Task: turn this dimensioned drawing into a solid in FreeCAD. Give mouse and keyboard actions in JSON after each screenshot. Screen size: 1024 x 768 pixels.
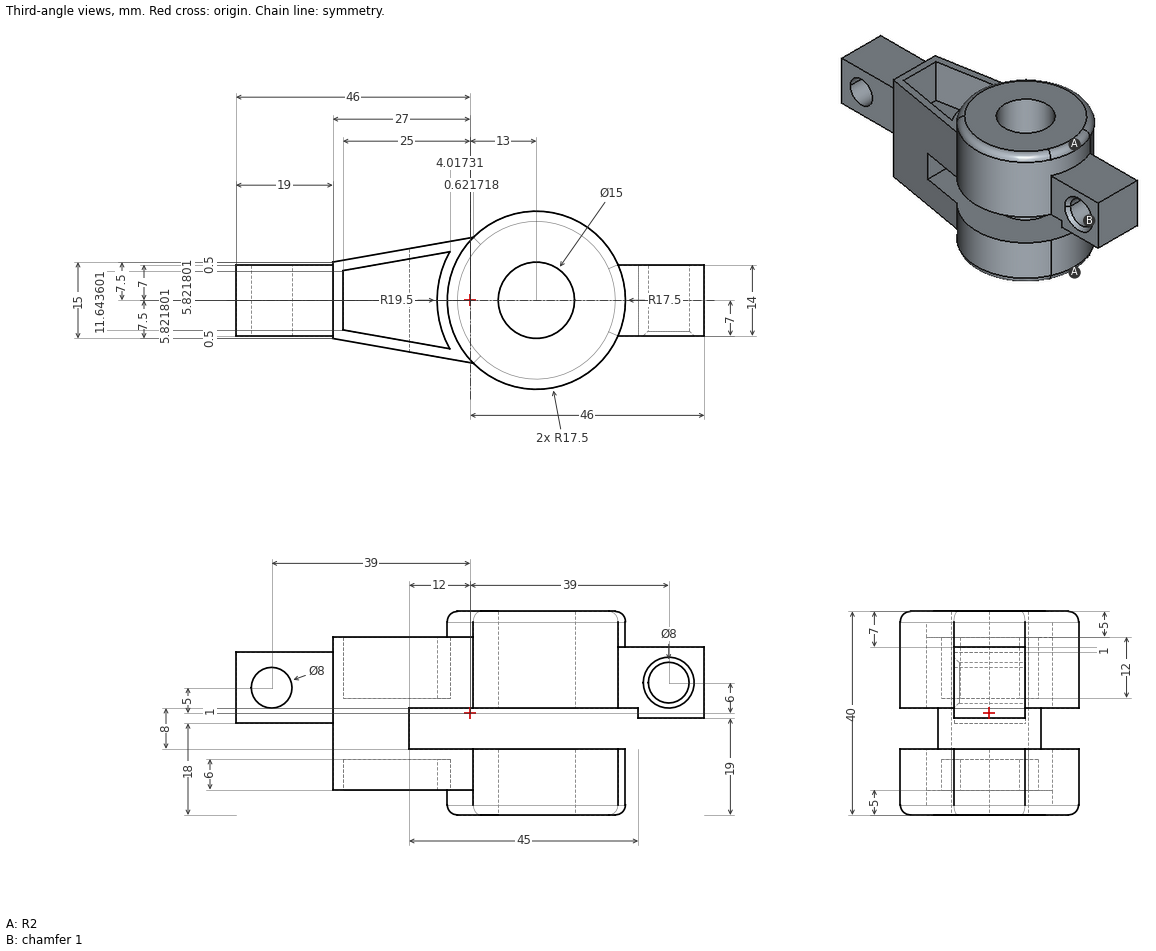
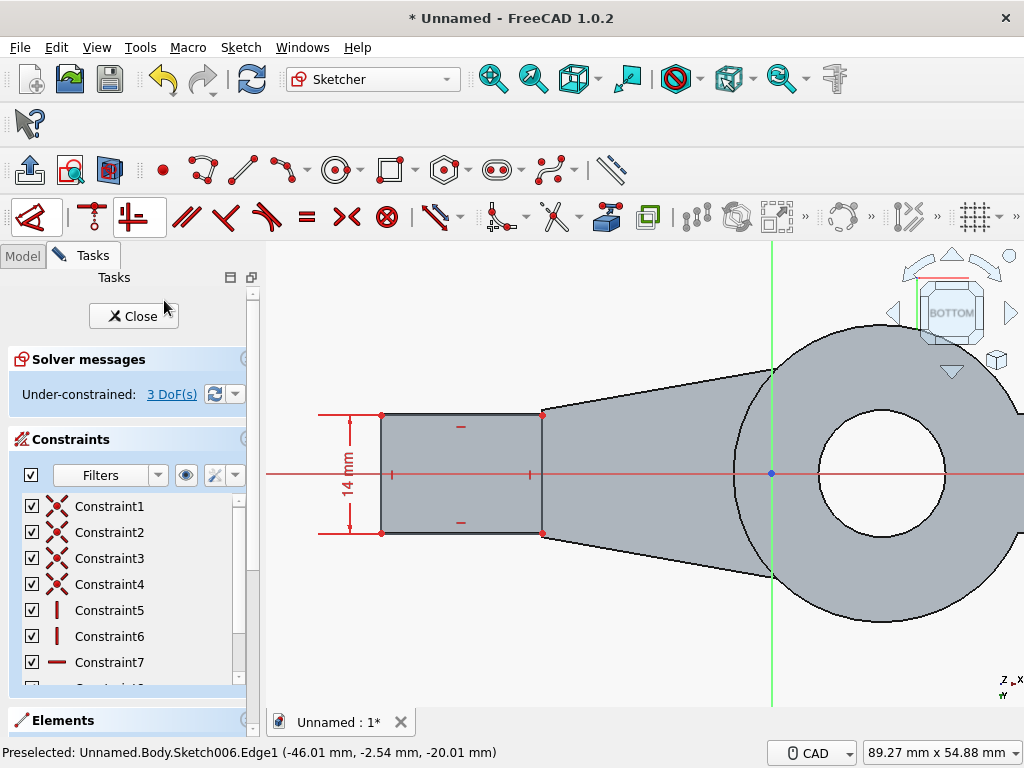
{"action": "left_click", "coordinate": [429, 534]}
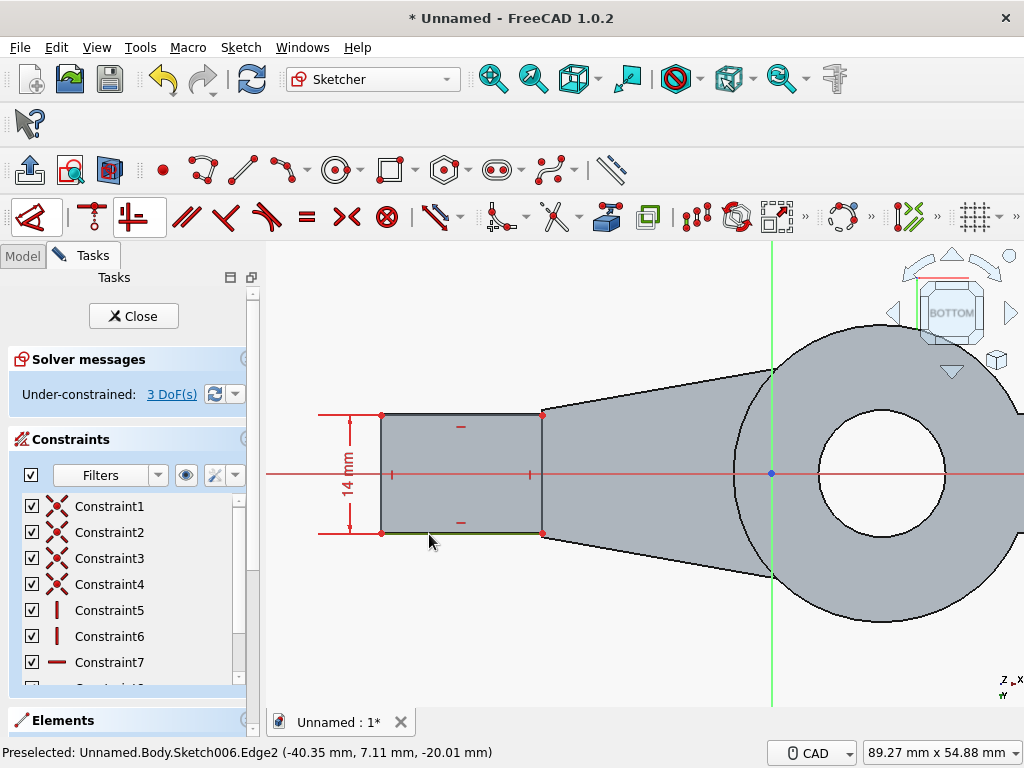
{"action": "left_click", "coordinate": [56, 218]}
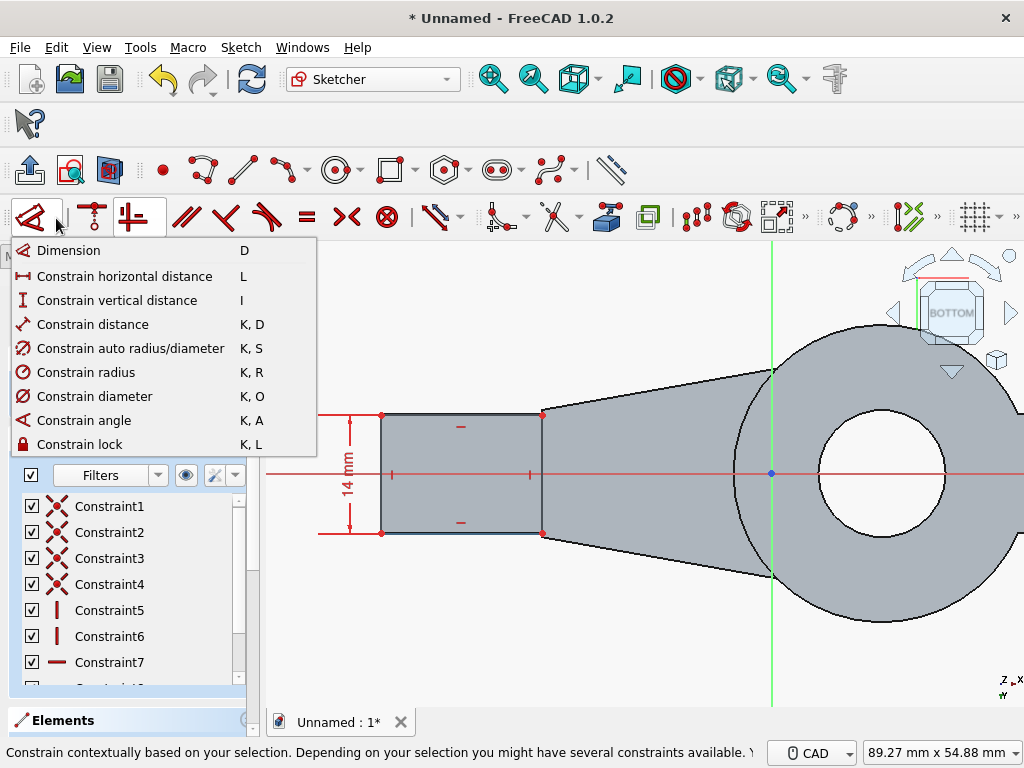
{"action": "left_click", "coordinate": [164, 276]}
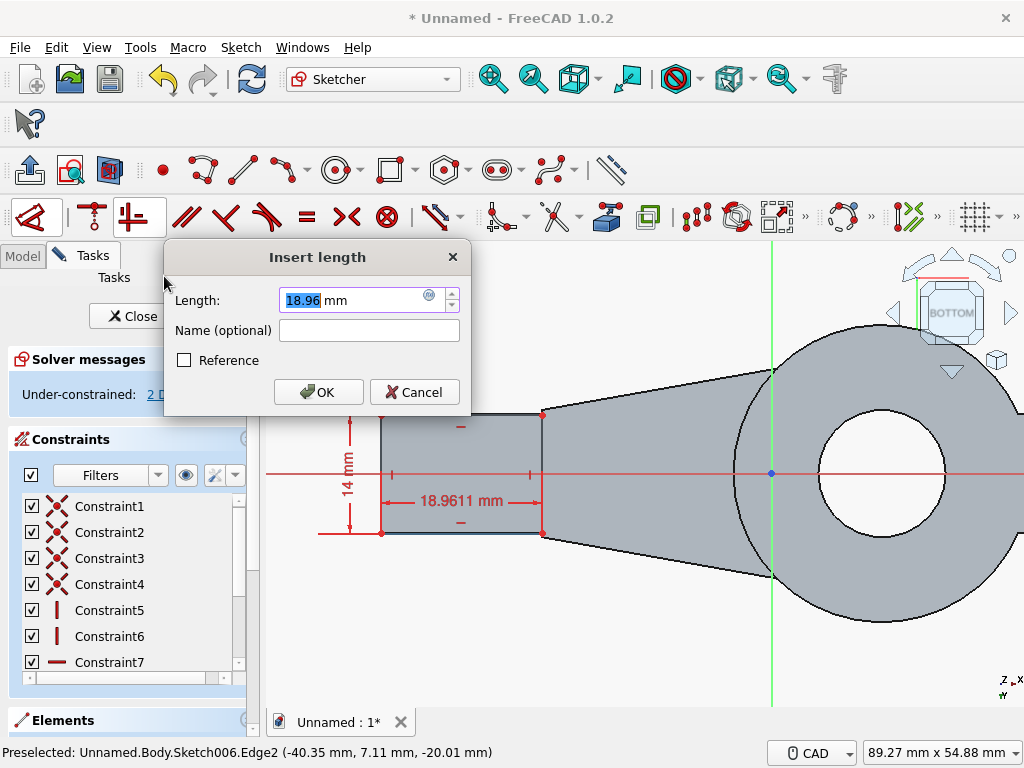
{"action": "type", "text": "19"}
{"action": "key", "text": "Return"}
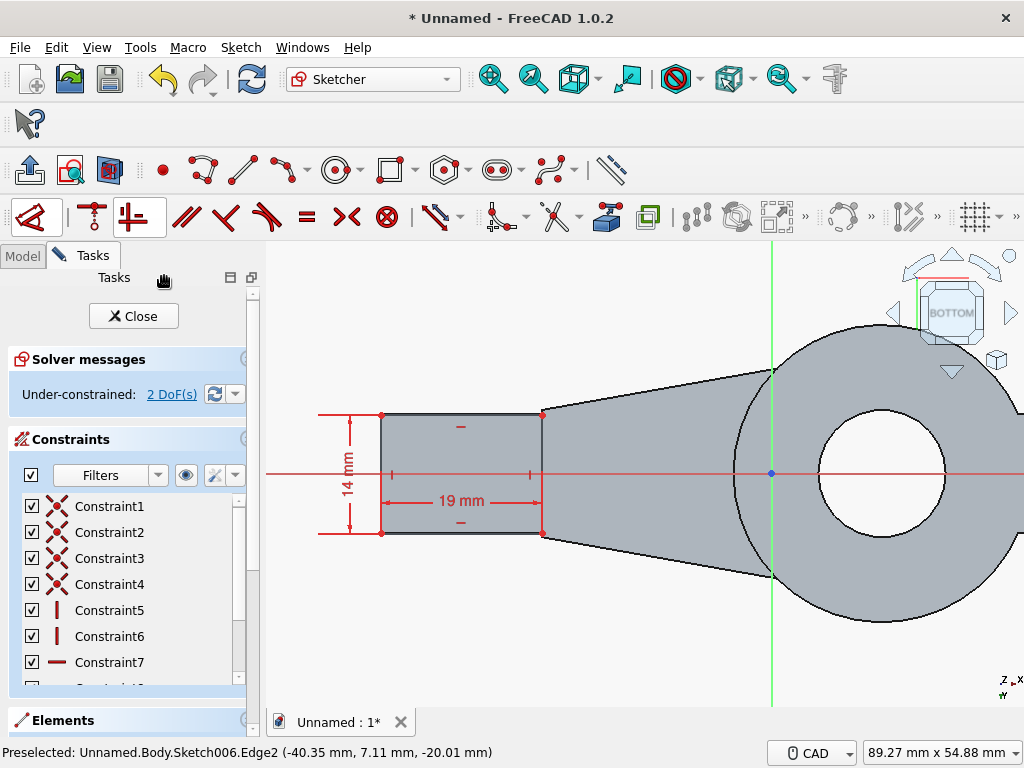
{"action": "left_click", "coordinate": [381, 415]}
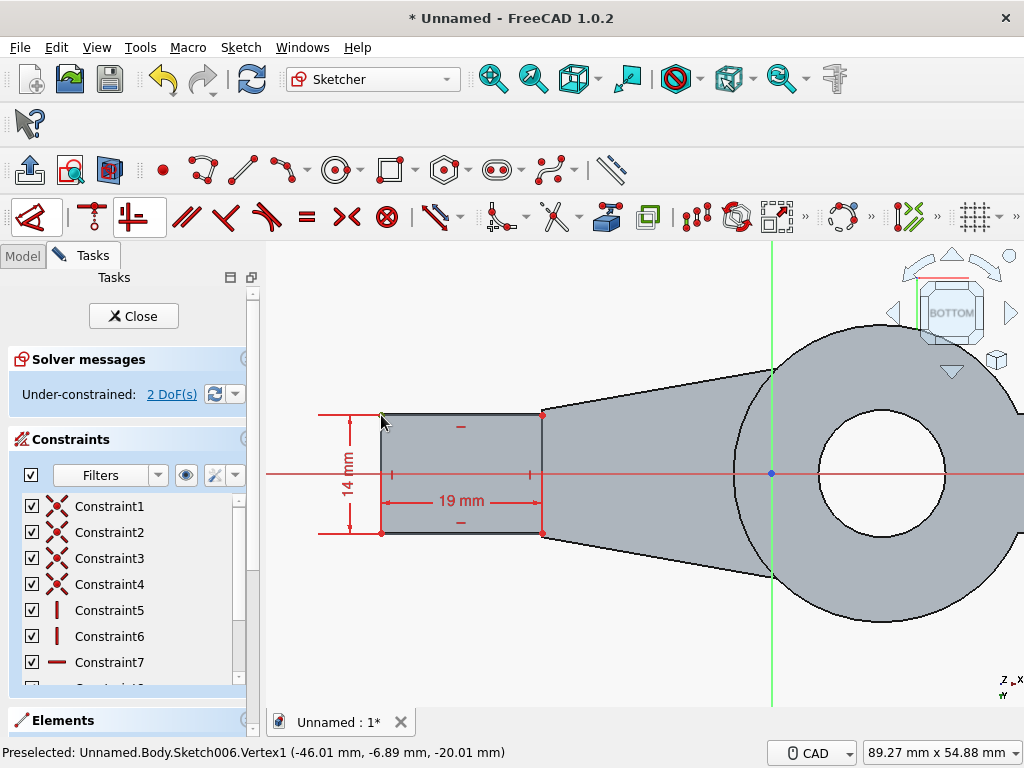
{"action": "left_click", "coordinate": [56, 218]}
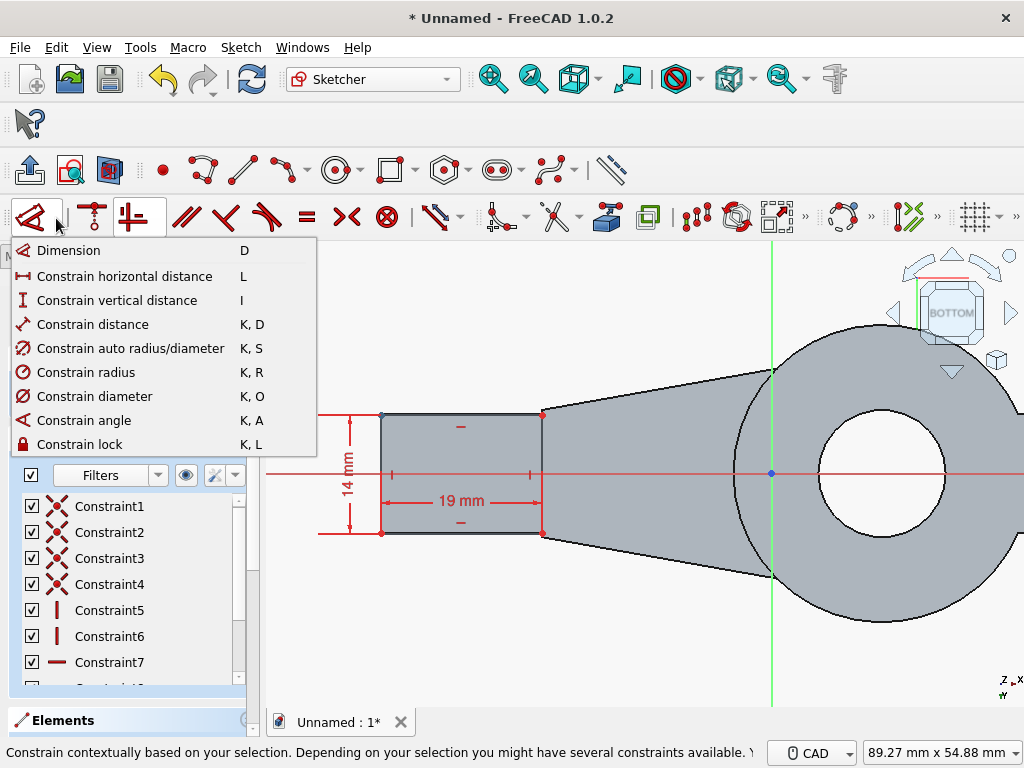
{"action": "left_click", "coordinate": [164, 300]}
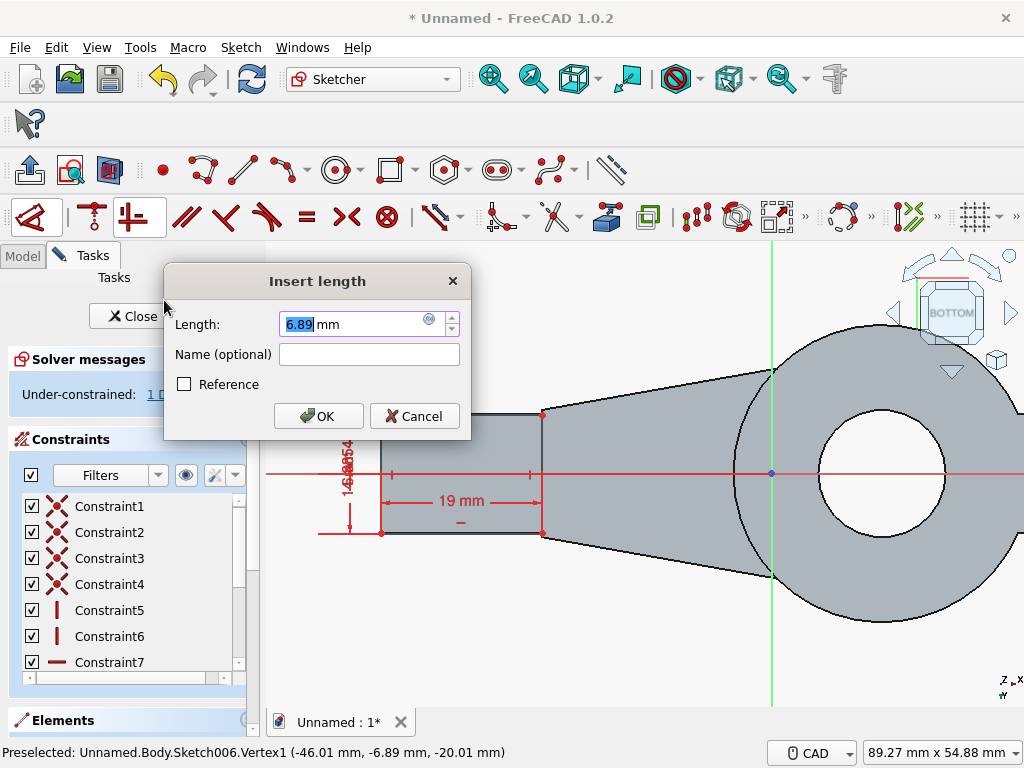
{"action": "type", "text": "7"}
{"action": "key", "text": "Return"}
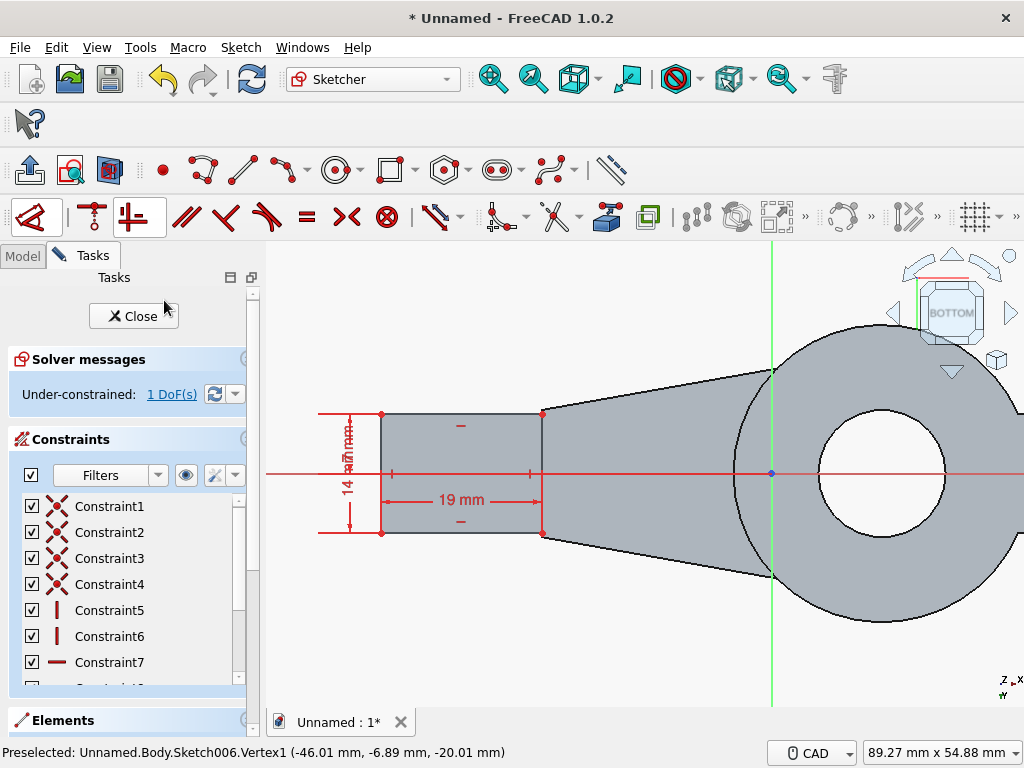
{"action": "left_click", "coordinate": [381, 414]}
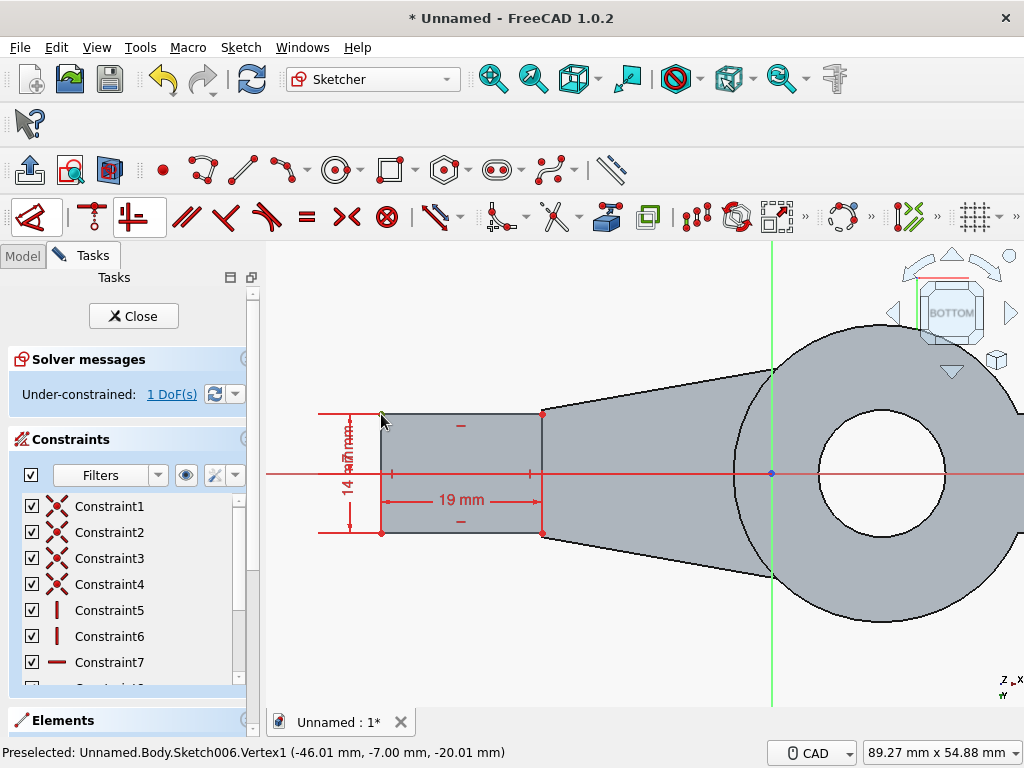
{"action": "key", "text": "l"}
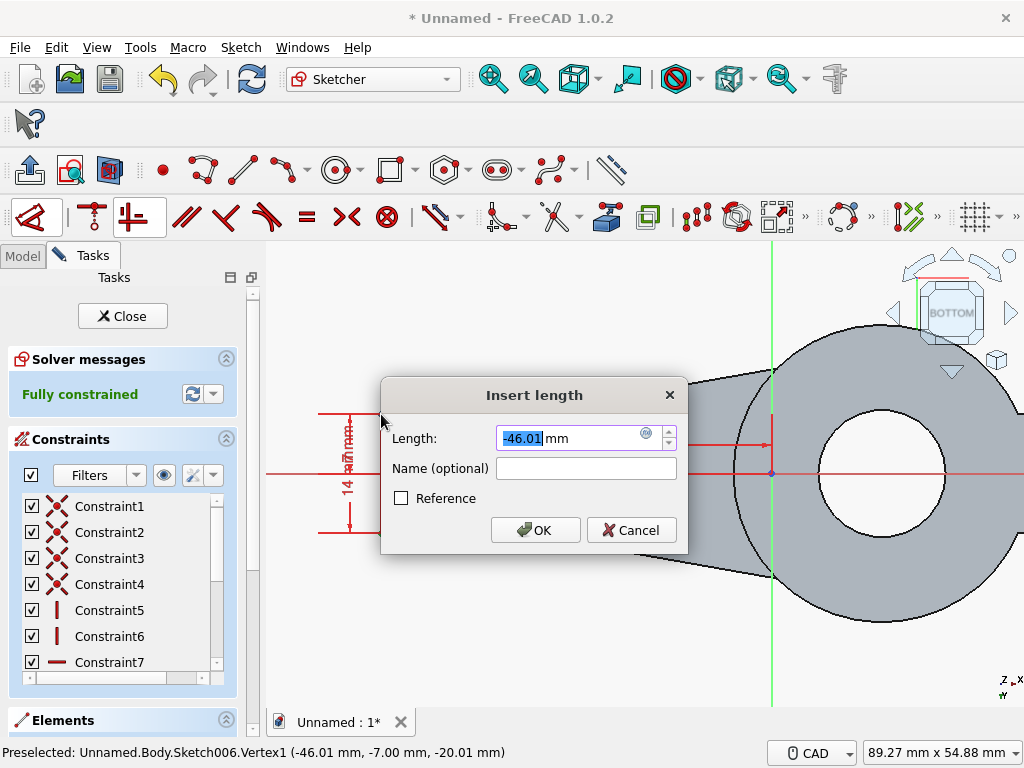
{"action": "type", "text": "-46"}
{"action": "key", "text": "Return"}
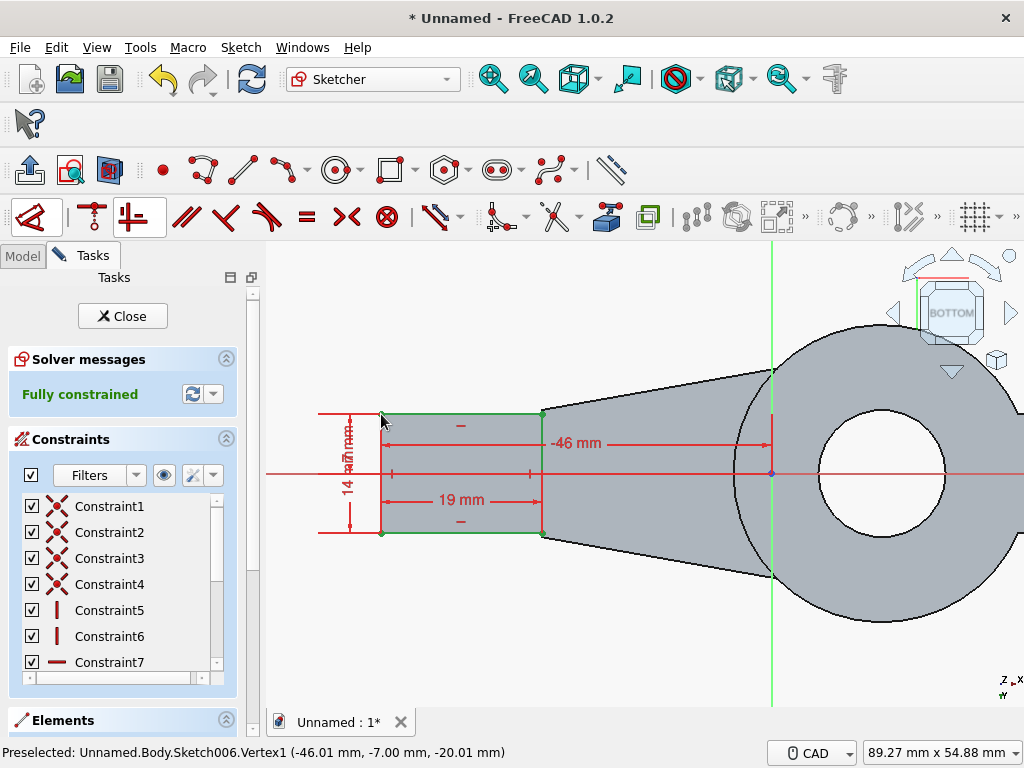
{"action": "left_click", "coordinate": [123, 316]}